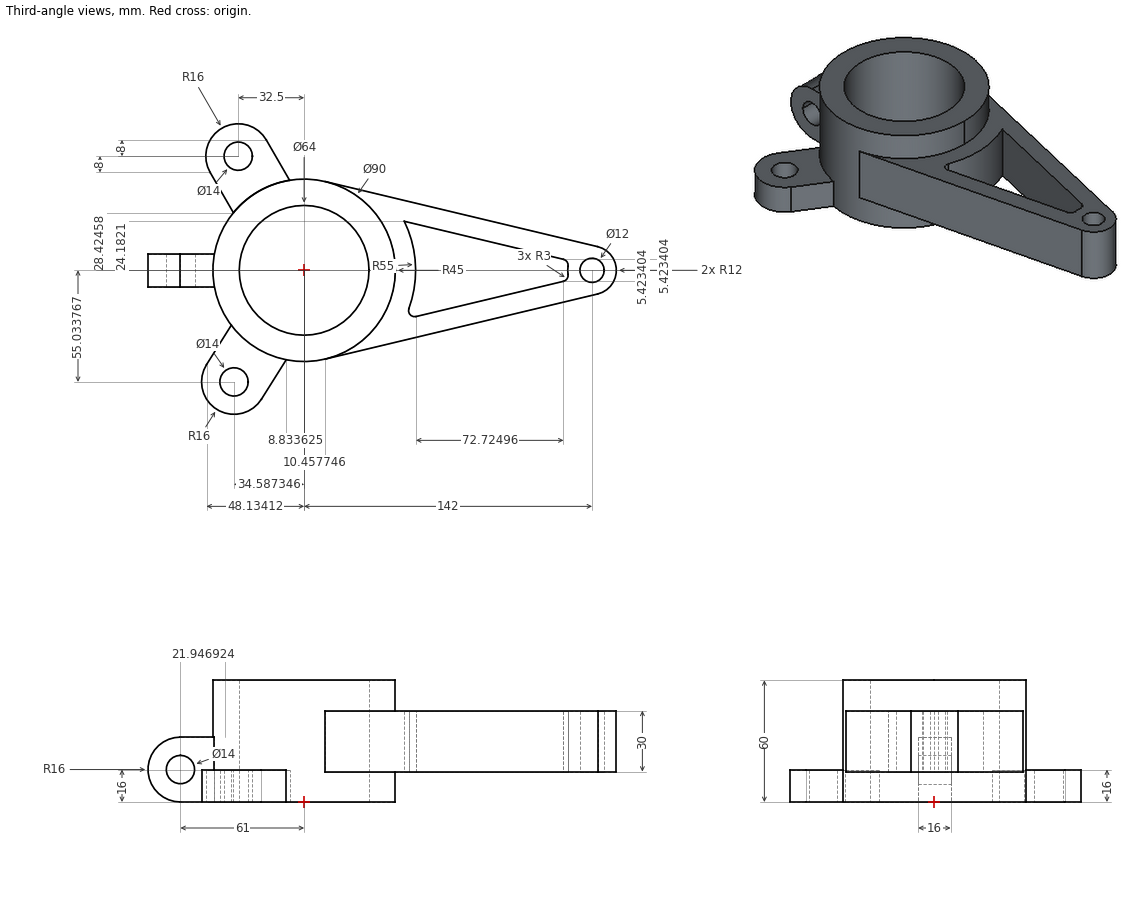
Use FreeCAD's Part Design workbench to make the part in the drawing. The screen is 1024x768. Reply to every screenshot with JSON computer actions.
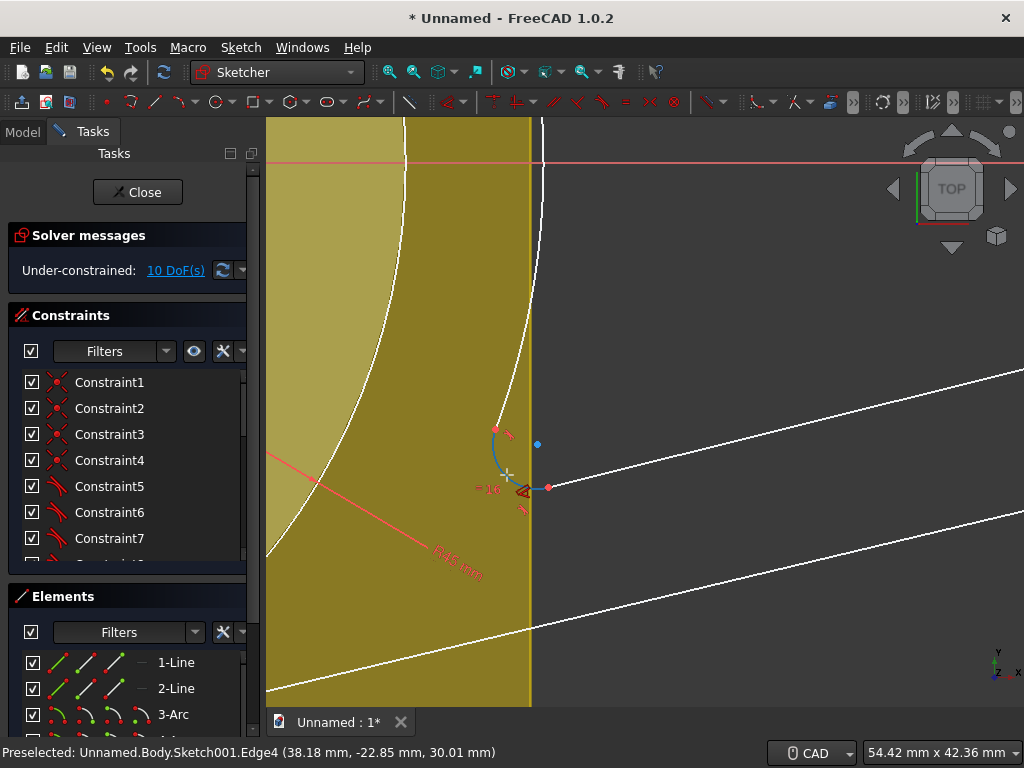
{"action": "left_click", "coordinate": [504, 474]}
{"action": "left_click", "coordinate": [480, 495]}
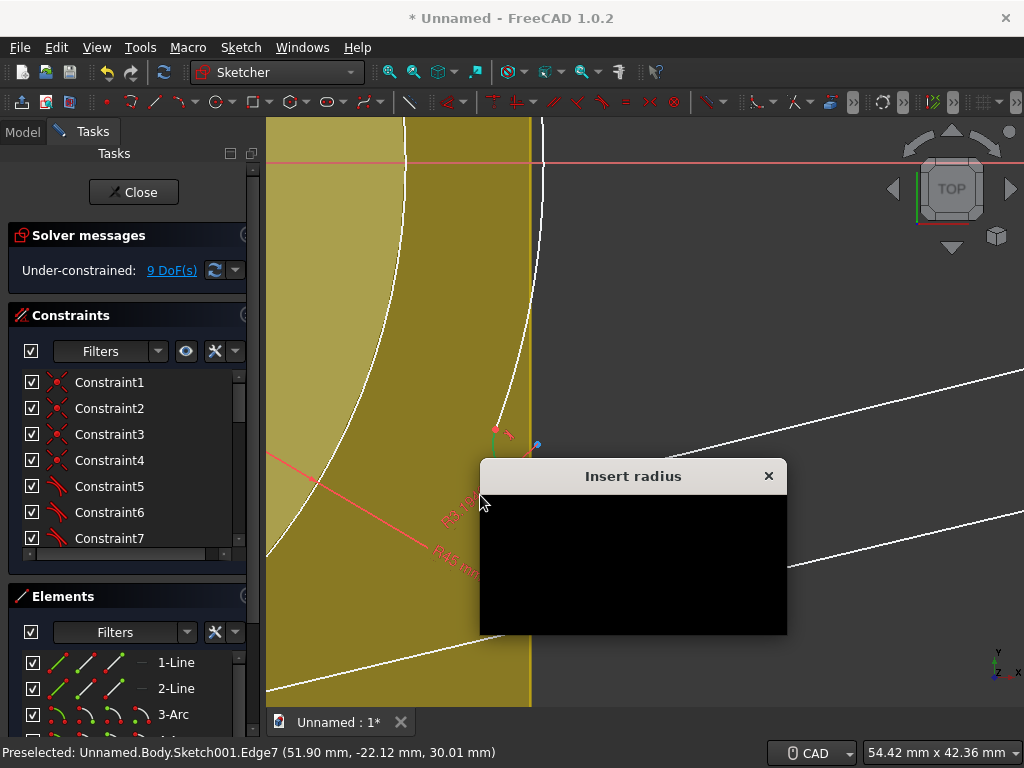
{"action": "type", "text": "3"}
{"action": "key", "text": "Return"}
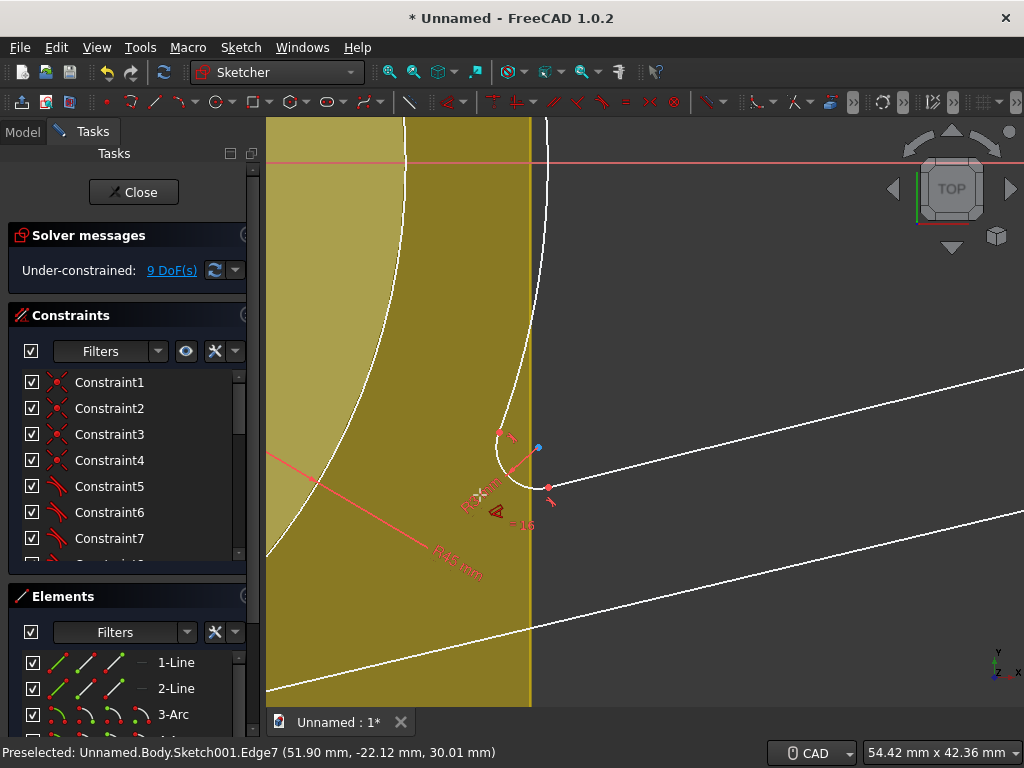
{"action": "scroll", "coordinate": [507, 475], "scroll_direction": "down", "scroll_amount": 8}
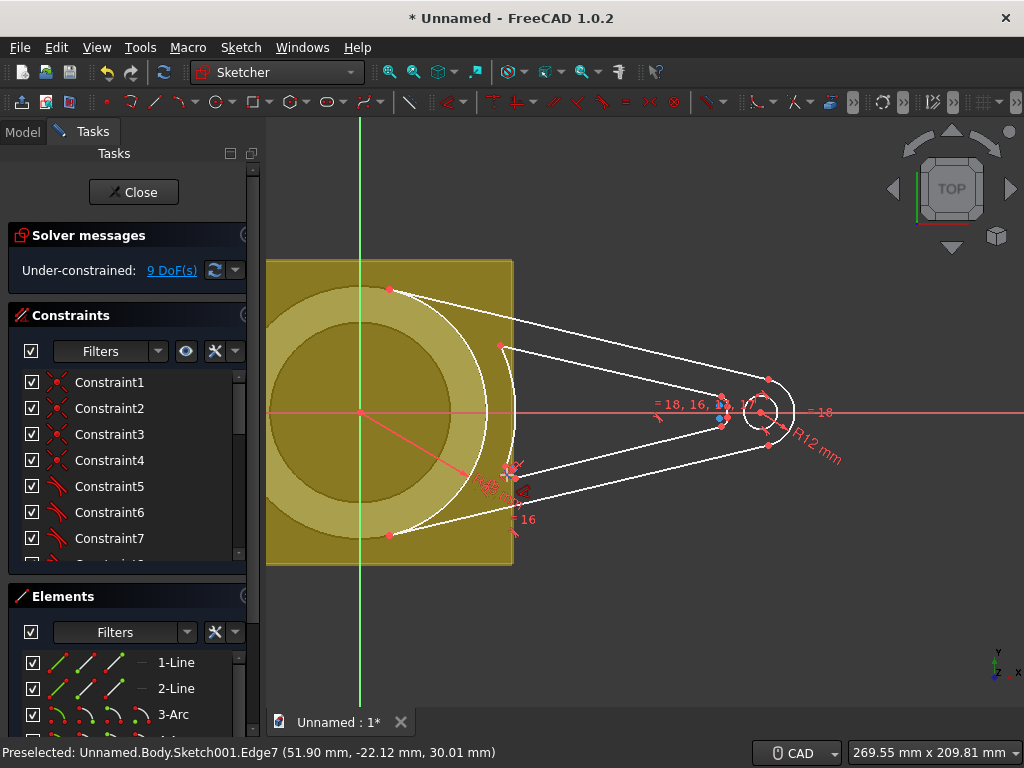
{"action": "left_click", "coordinate": [514, 431]}
{"action": "left_click", "coordinate": [546, 435]}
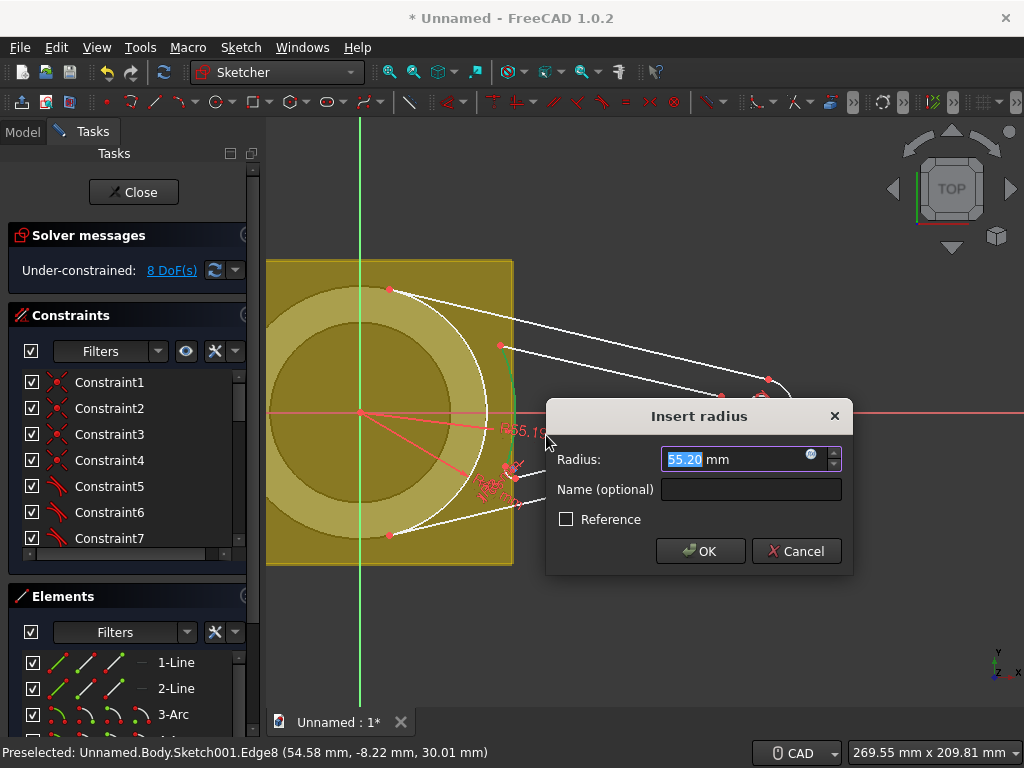
{"action": "type", "text": "55"}
{"action": "key", "text": "Return"}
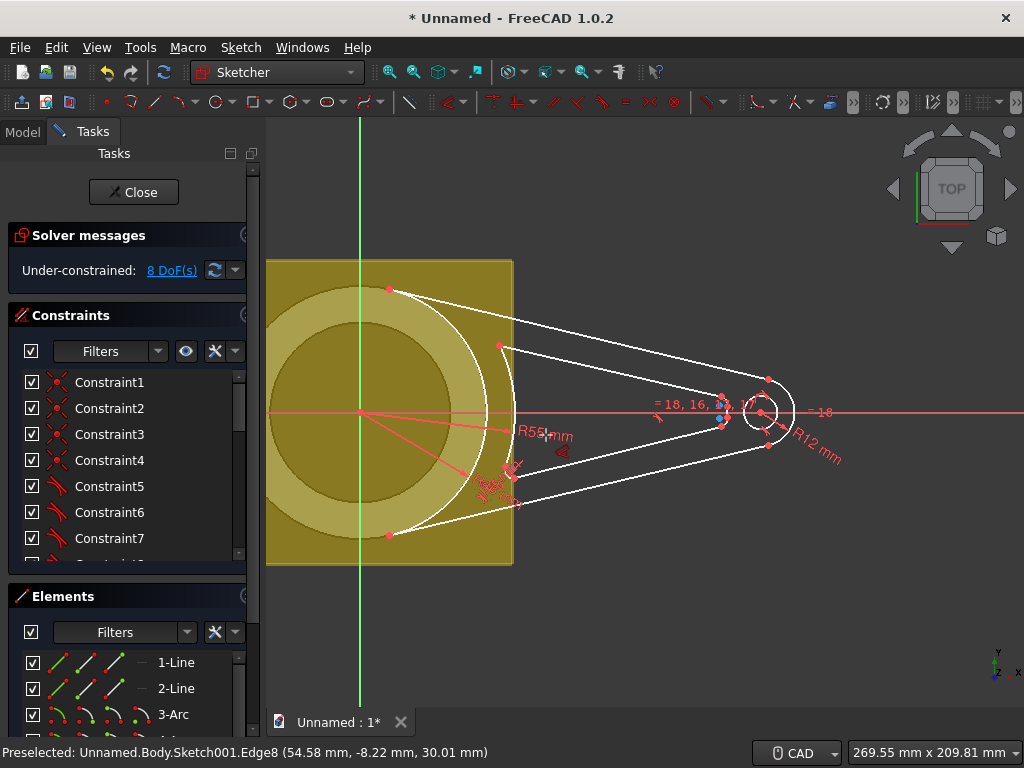
{"action": "left_click", "coordinate": [773, 401]}
{"action": "left_click", "coordinate": [796, 379]}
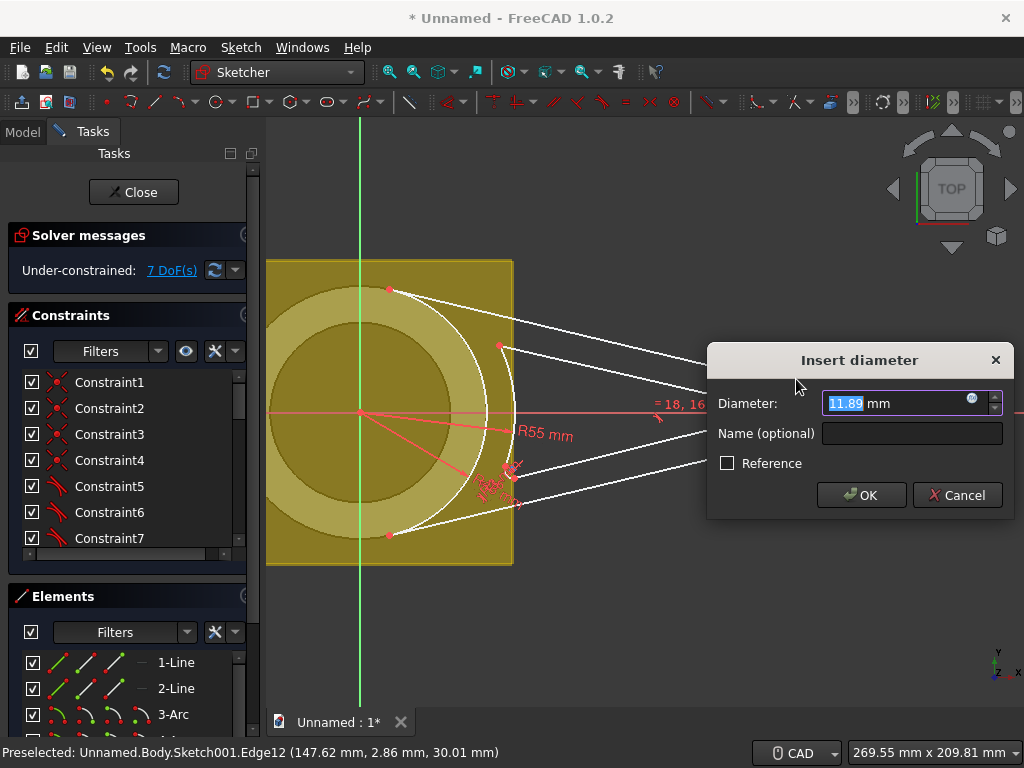
{"action": "type", "text": "12"}
{"action": "key", "text": "Return"}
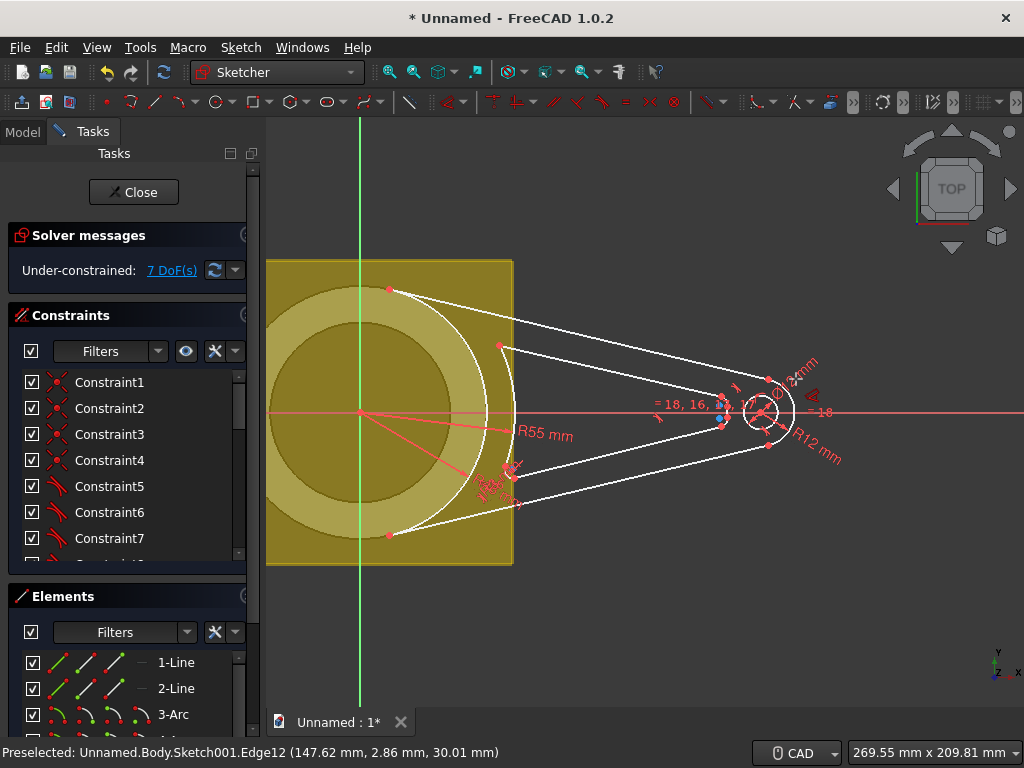
{"action": "left_click", "coordinate": [761, 413]}
{"action": "left_click", "coordinate": [468, 447]}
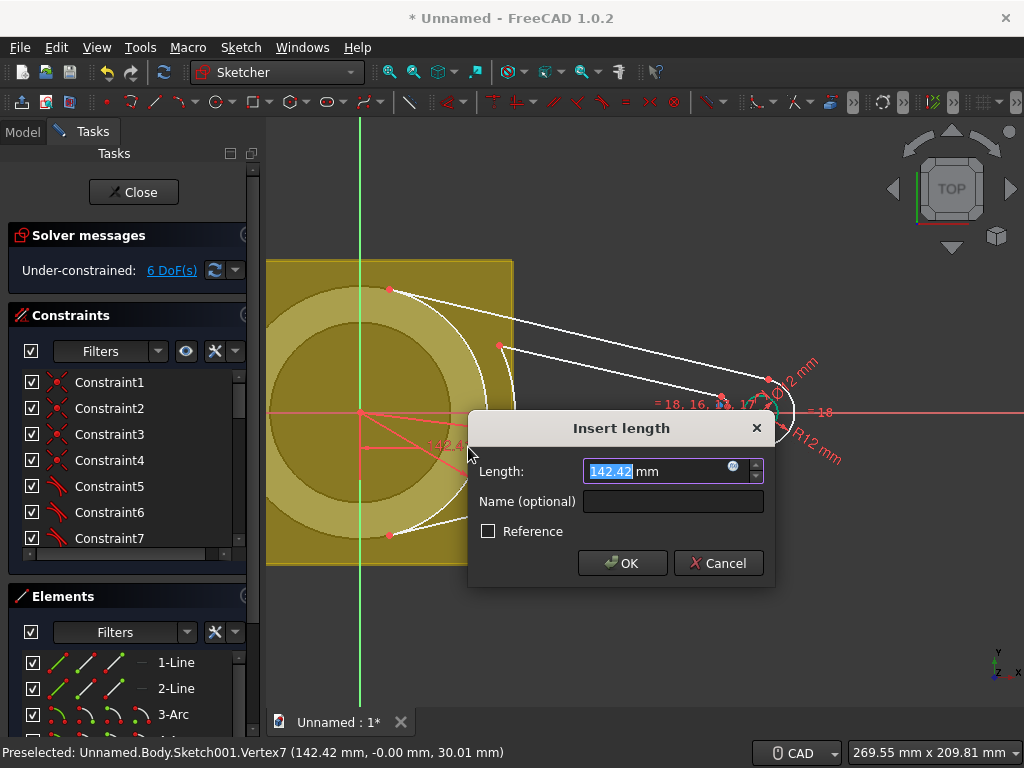
{"action": "type", "text": "142"}
{"action": "key", "text": "Return"}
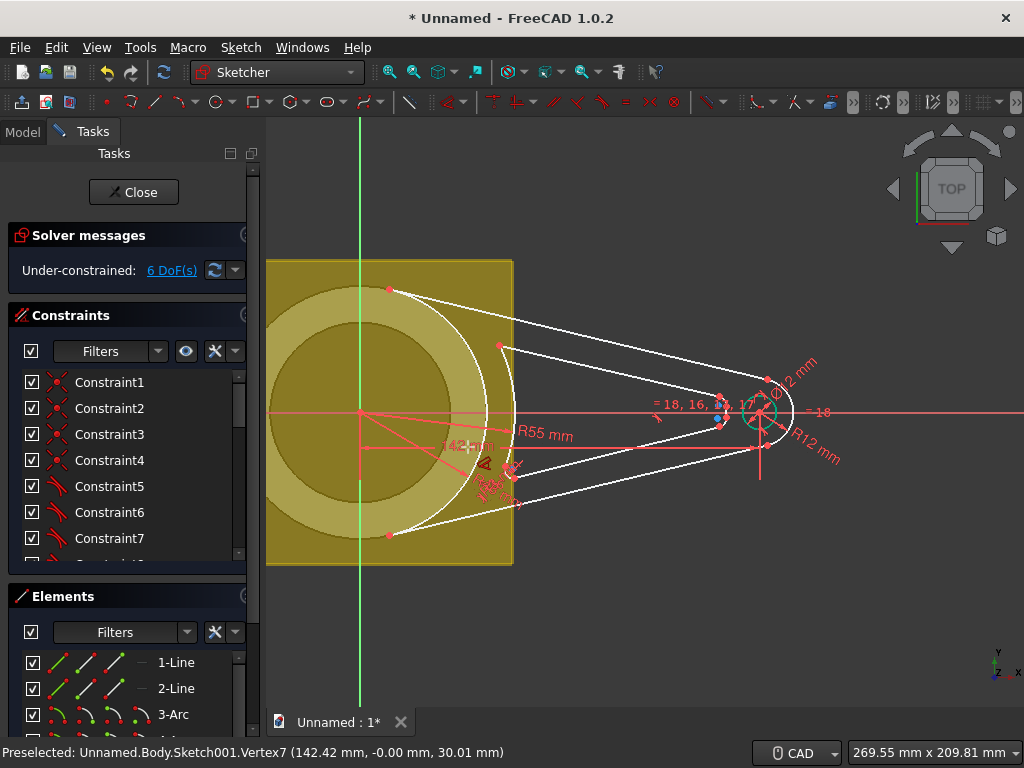
{"action": "left_click", "coordinate": [500, 346]}
{"action": "left_click", "coordinate": [326, 379]}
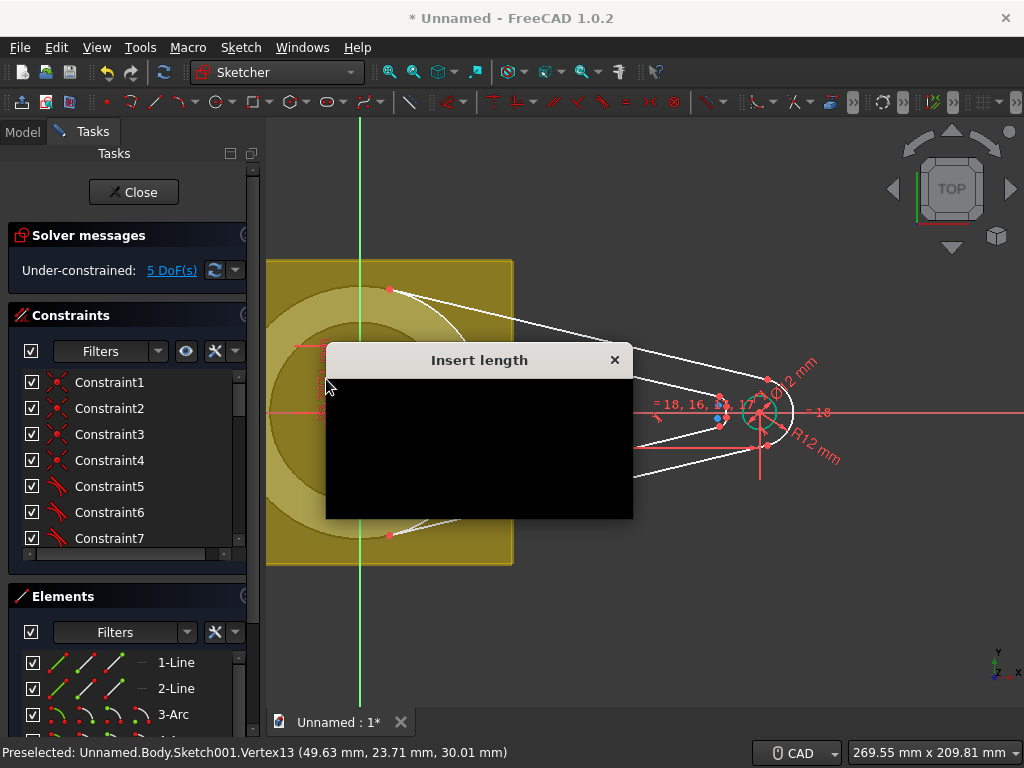
{"action": "type", "text": "24.1821"}
{"action": "key", "text": "Return"}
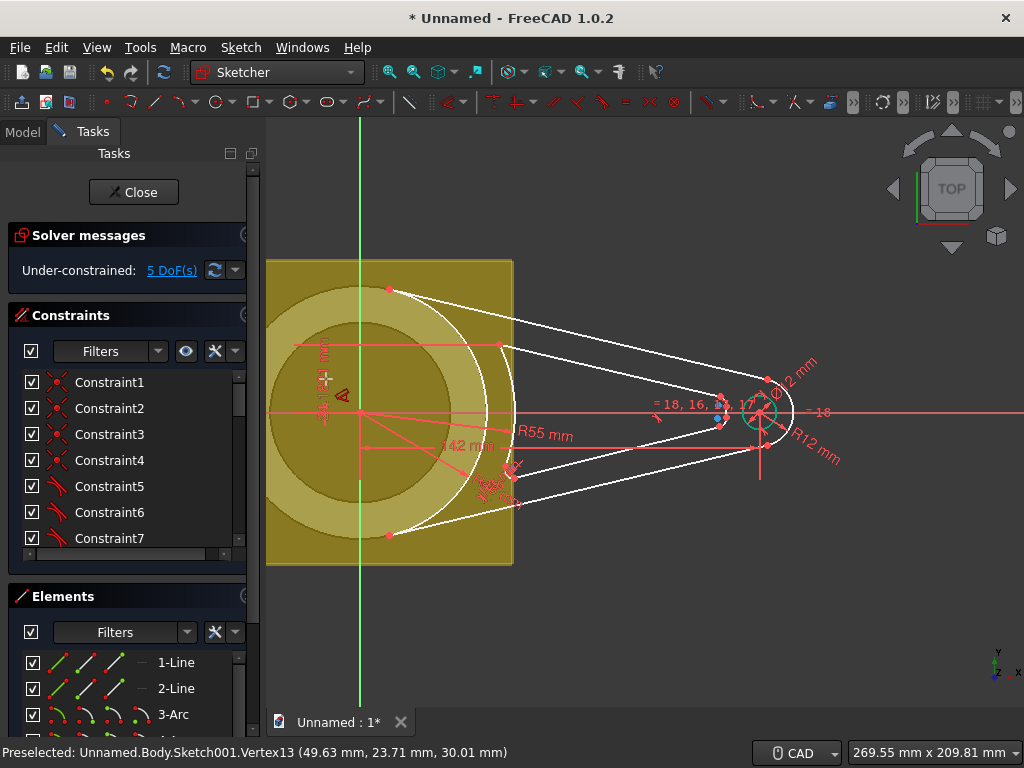
{"action": "scroll", "coordinate": [720, 427], "scroll_direction": "up", "scroll_amount": 5}